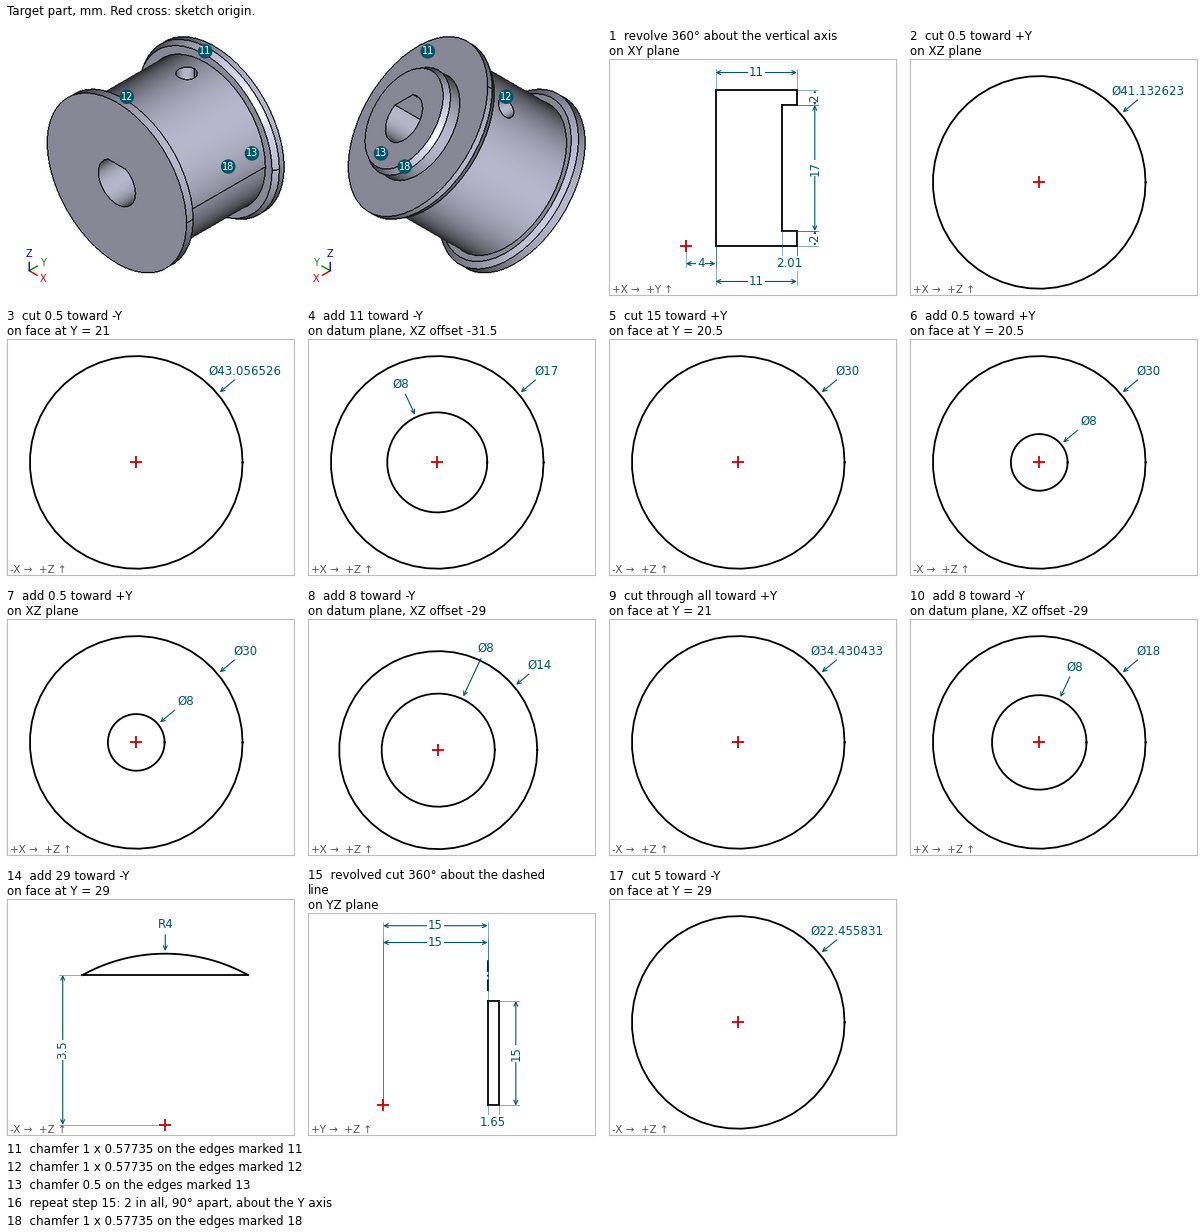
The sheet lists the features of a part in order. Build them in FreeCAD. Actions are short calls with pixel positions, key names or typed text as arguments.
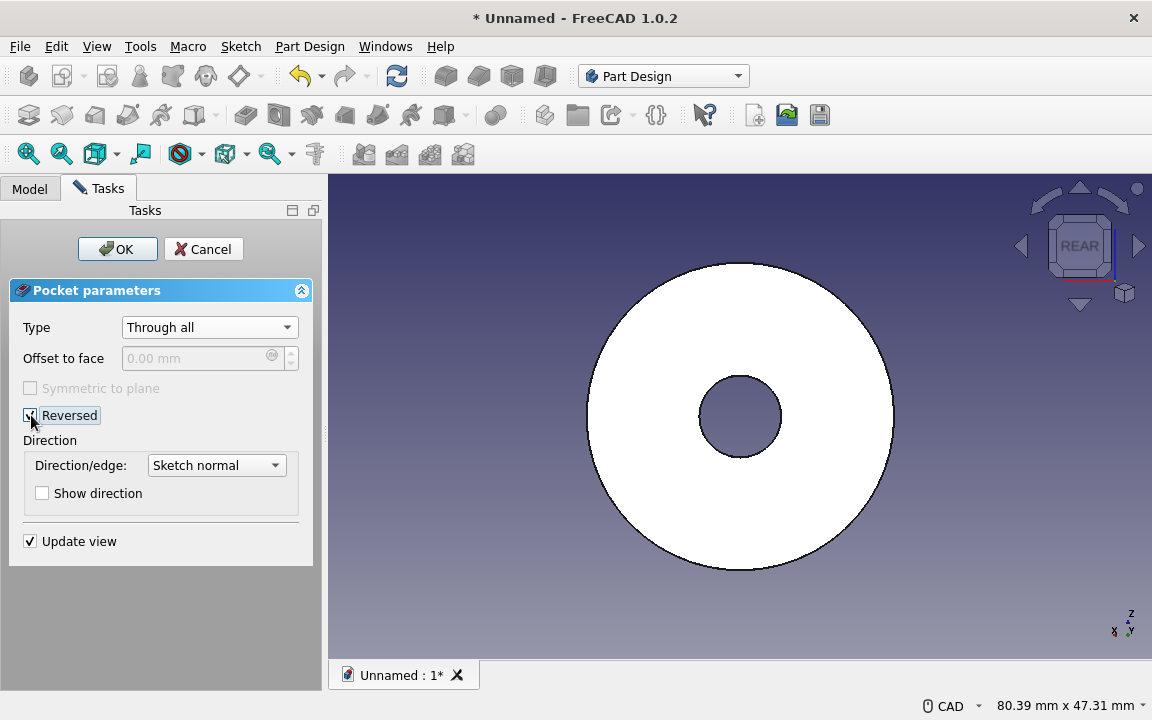
click(118, 249)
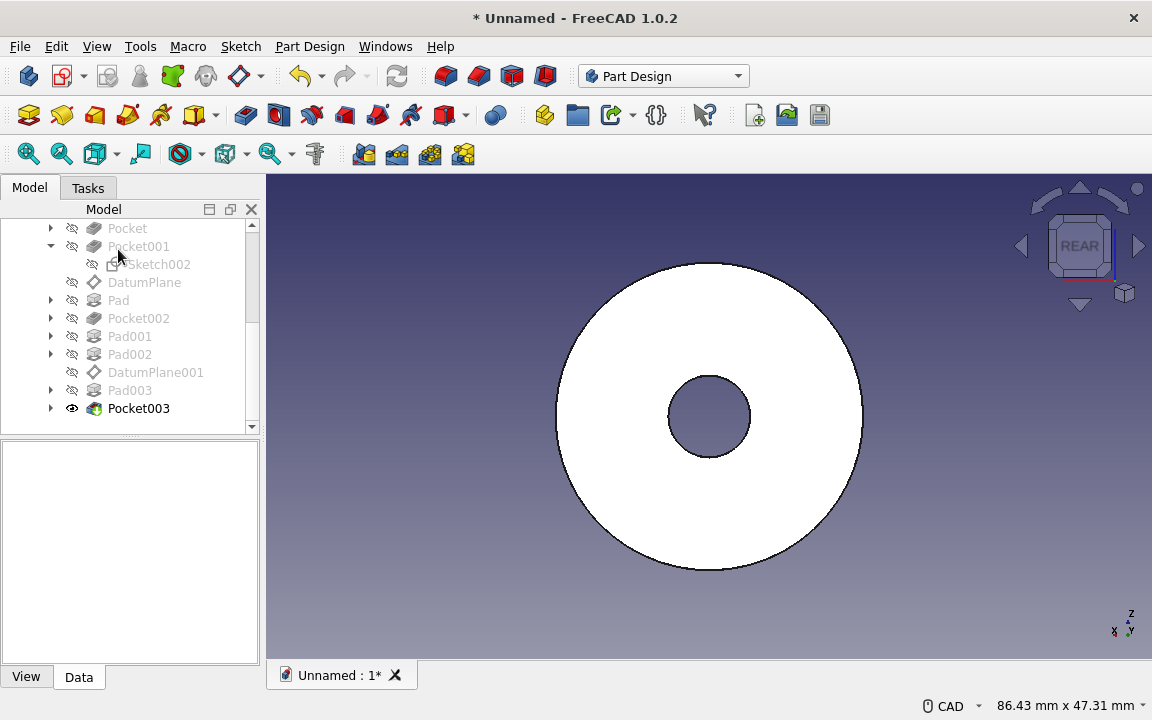
scroll(141, 314, down, 3)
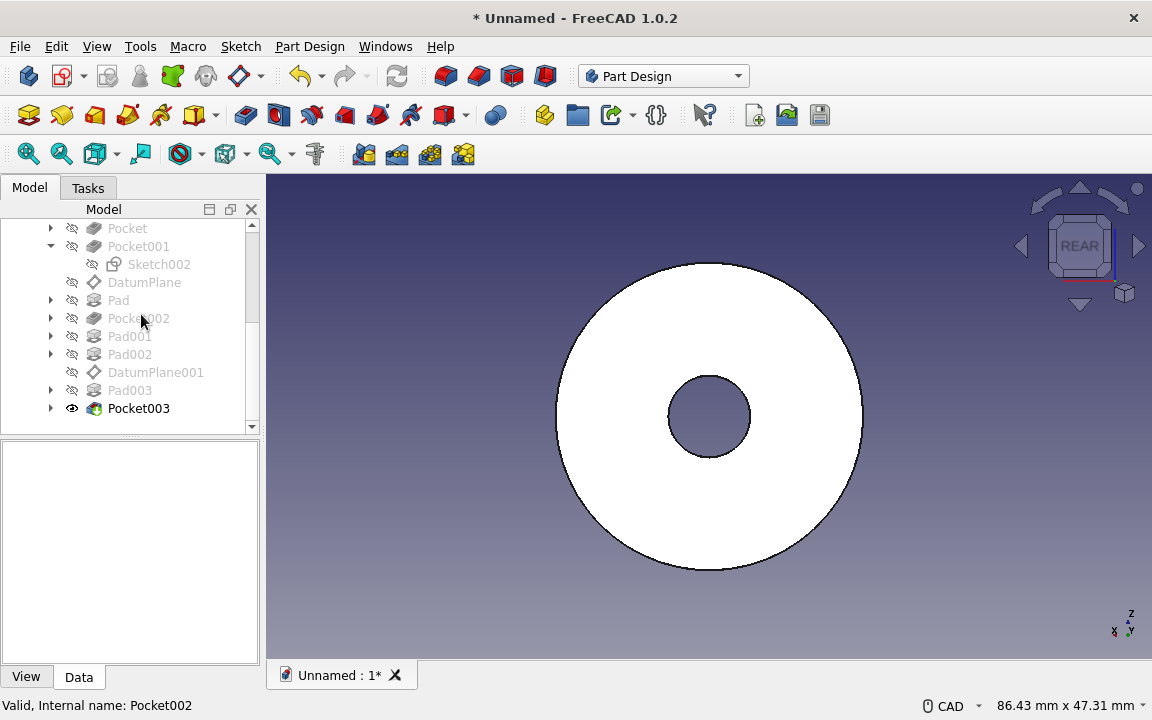
scroll(141, 314, up, 15)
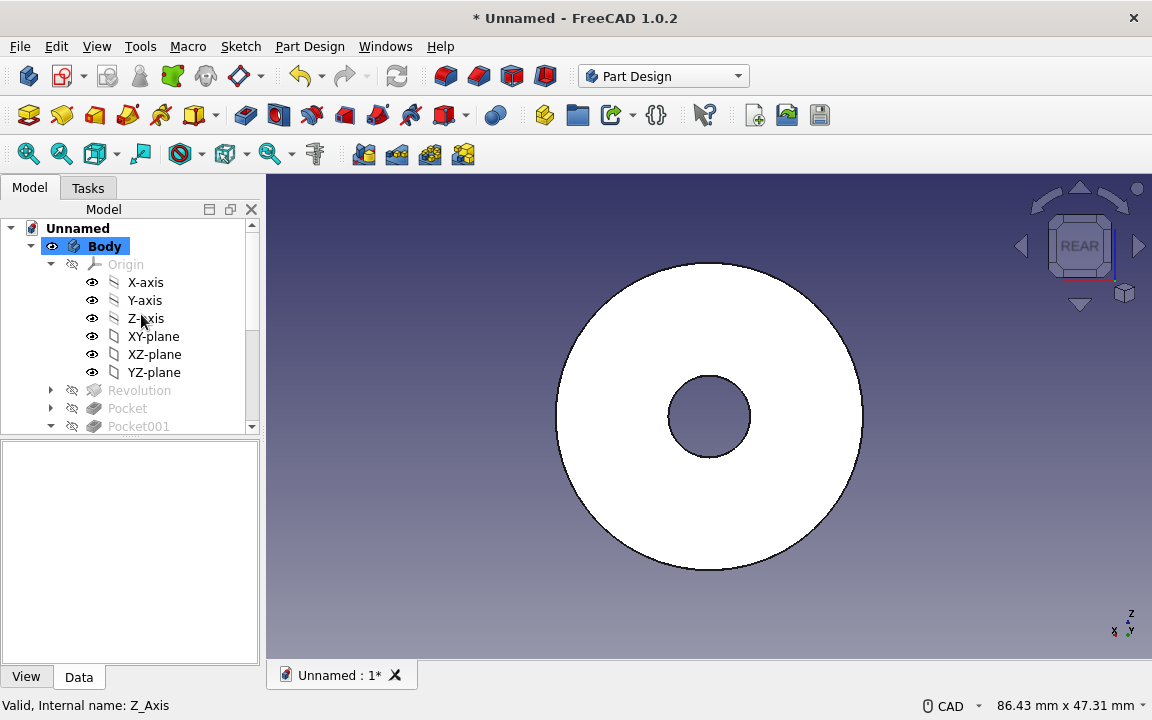
click(137, 354)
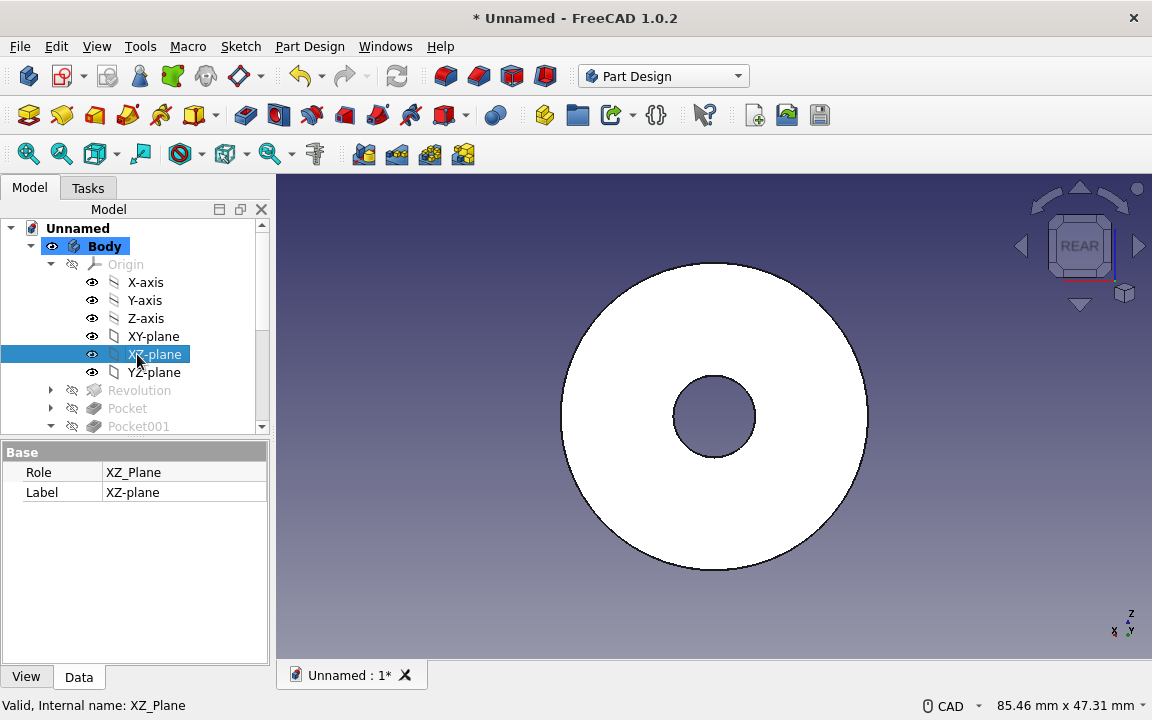
click(238, 76)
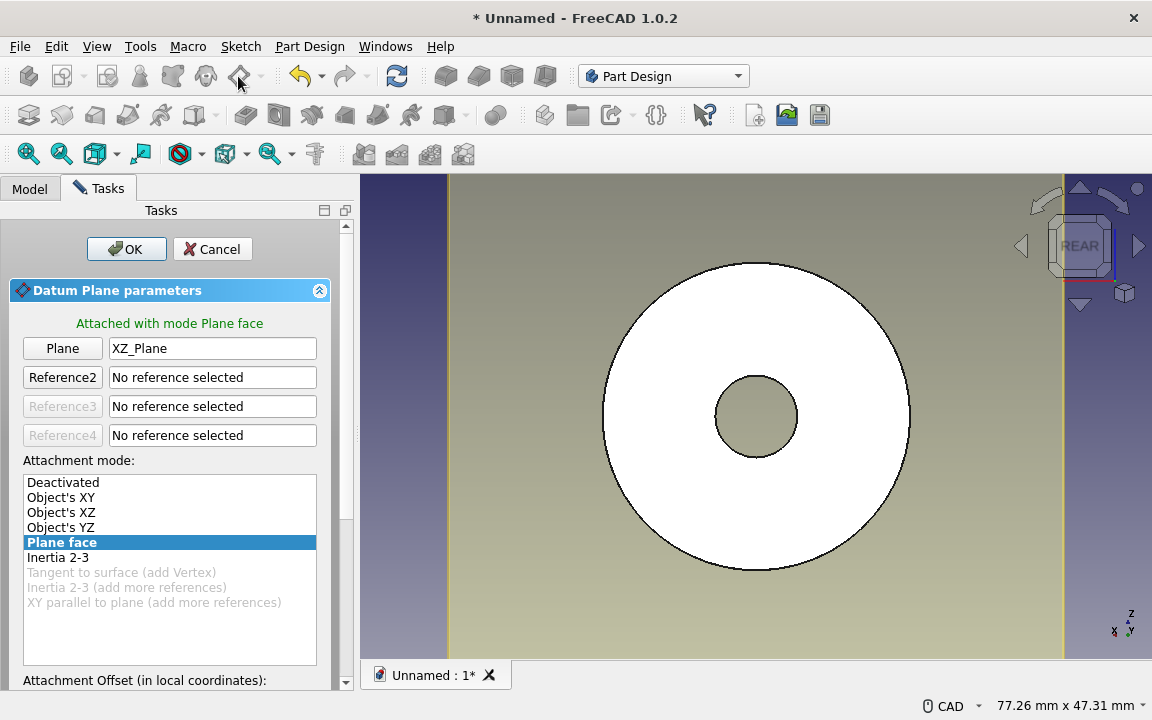
scroll(346, 455, down, 3)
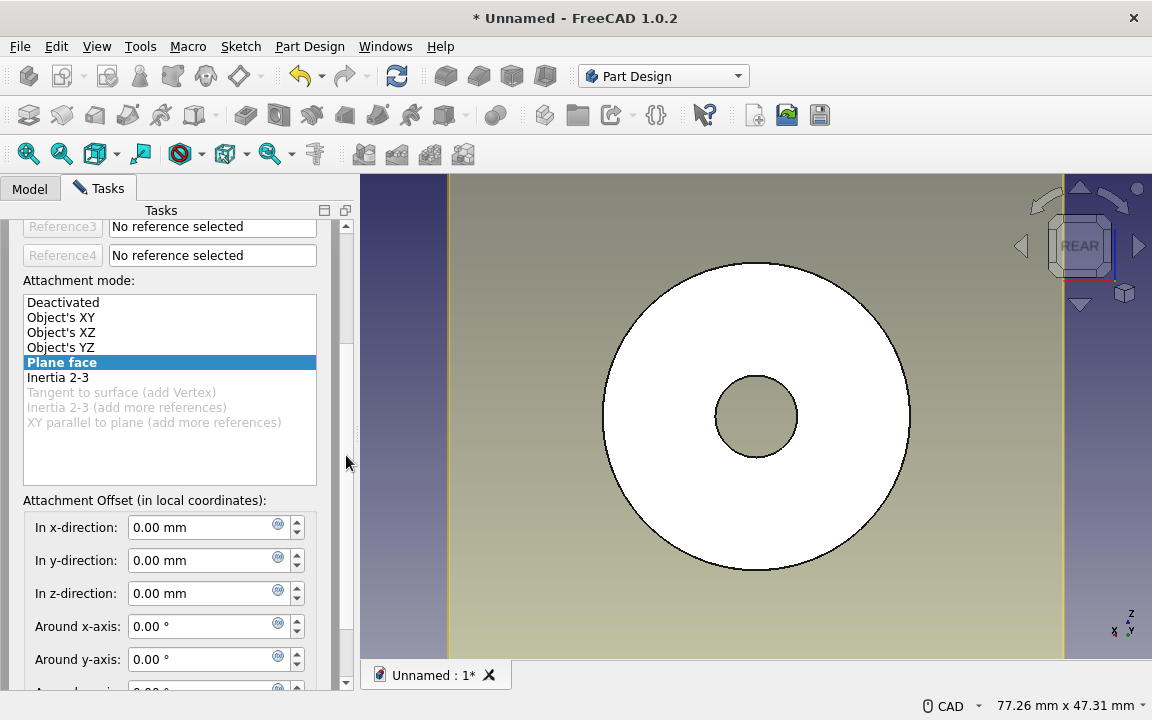
triple_click(210, 594)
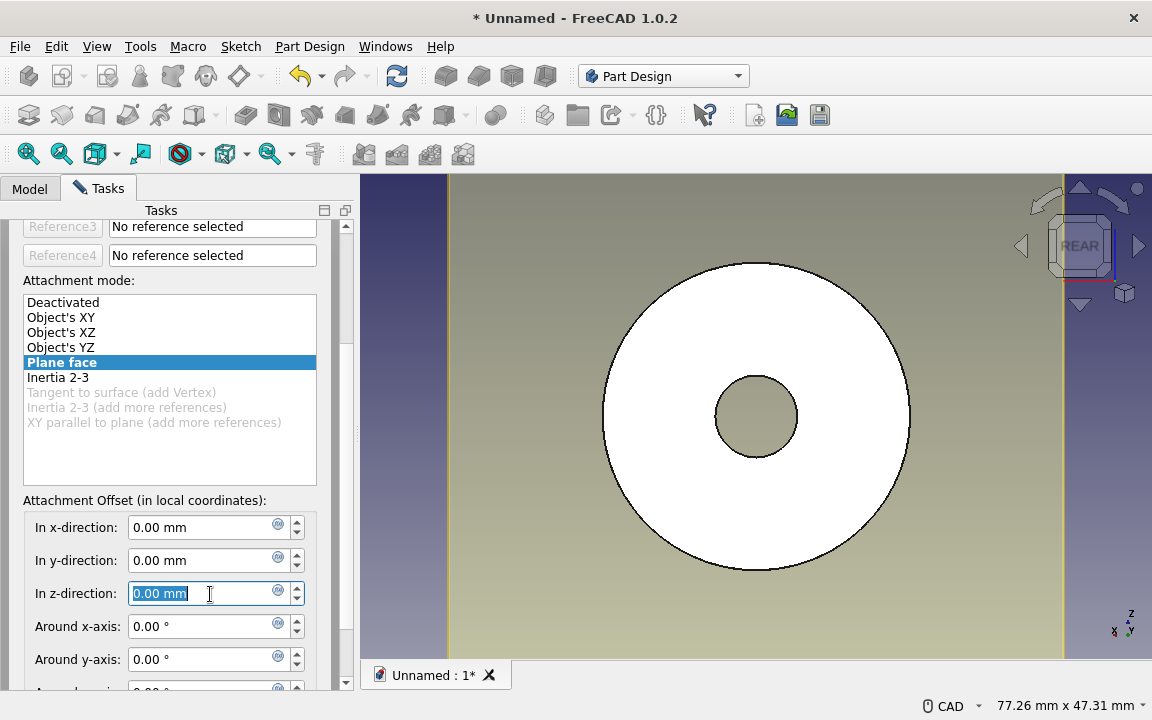
text(-29)
key(Tab)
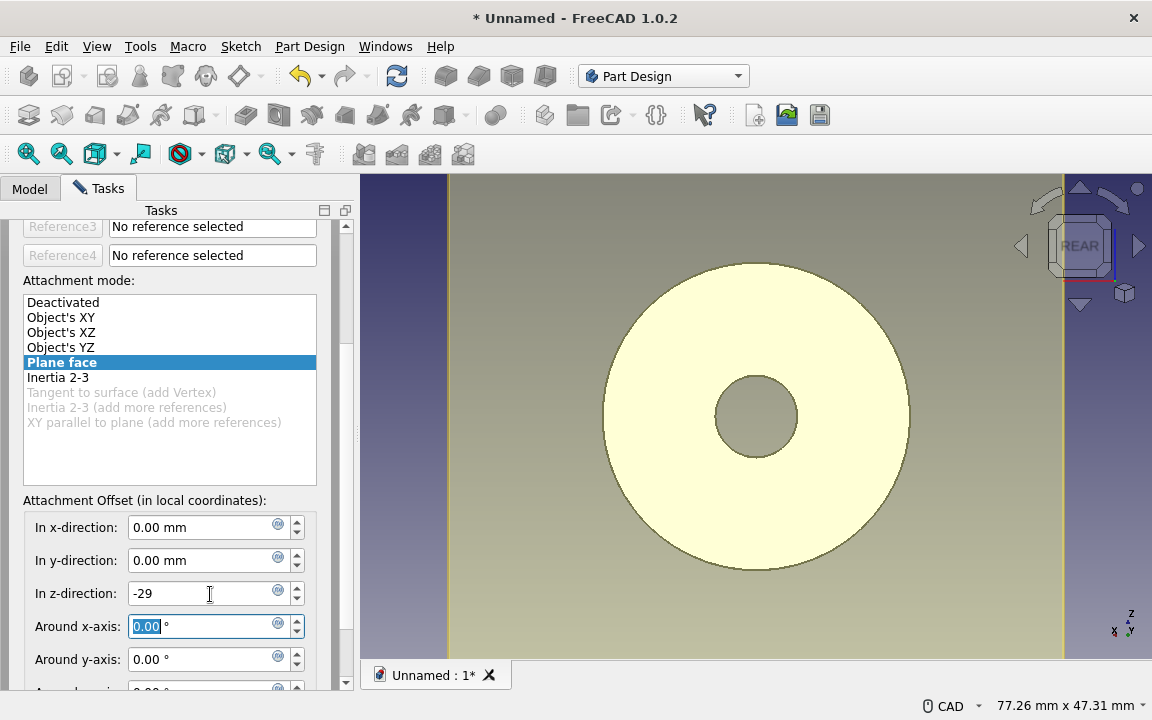
scroll(346, 455, up, 4)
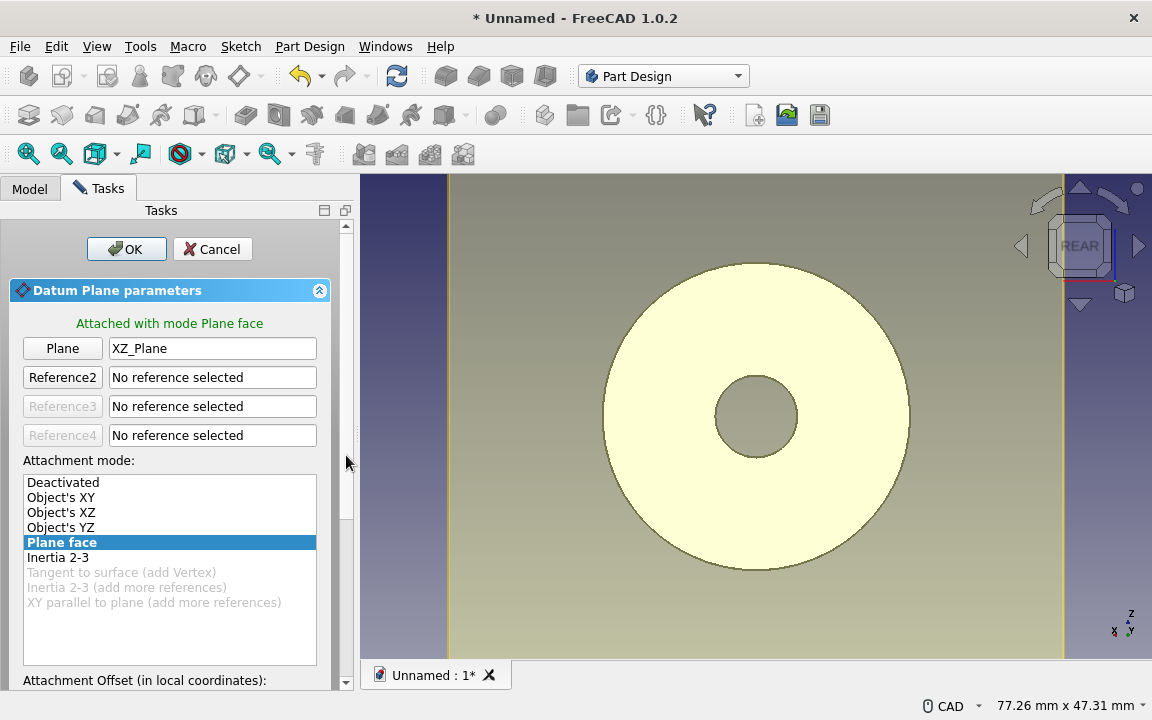
click(127, 249)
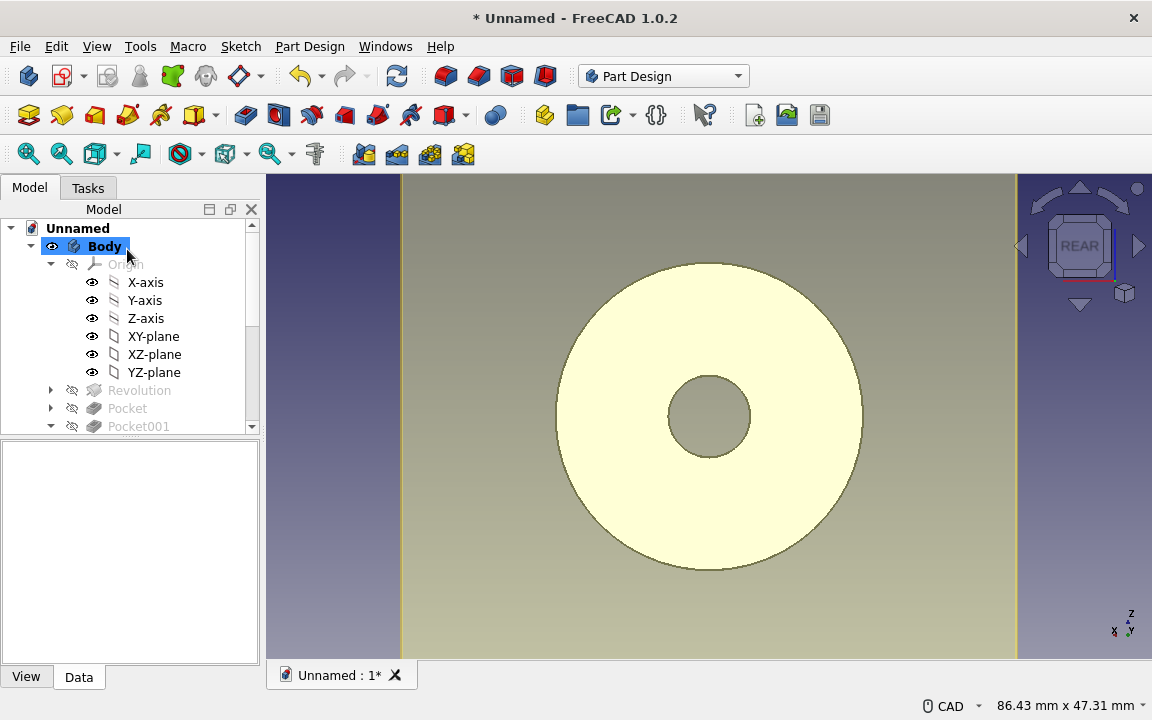
scroll(101, 332, down, 3)